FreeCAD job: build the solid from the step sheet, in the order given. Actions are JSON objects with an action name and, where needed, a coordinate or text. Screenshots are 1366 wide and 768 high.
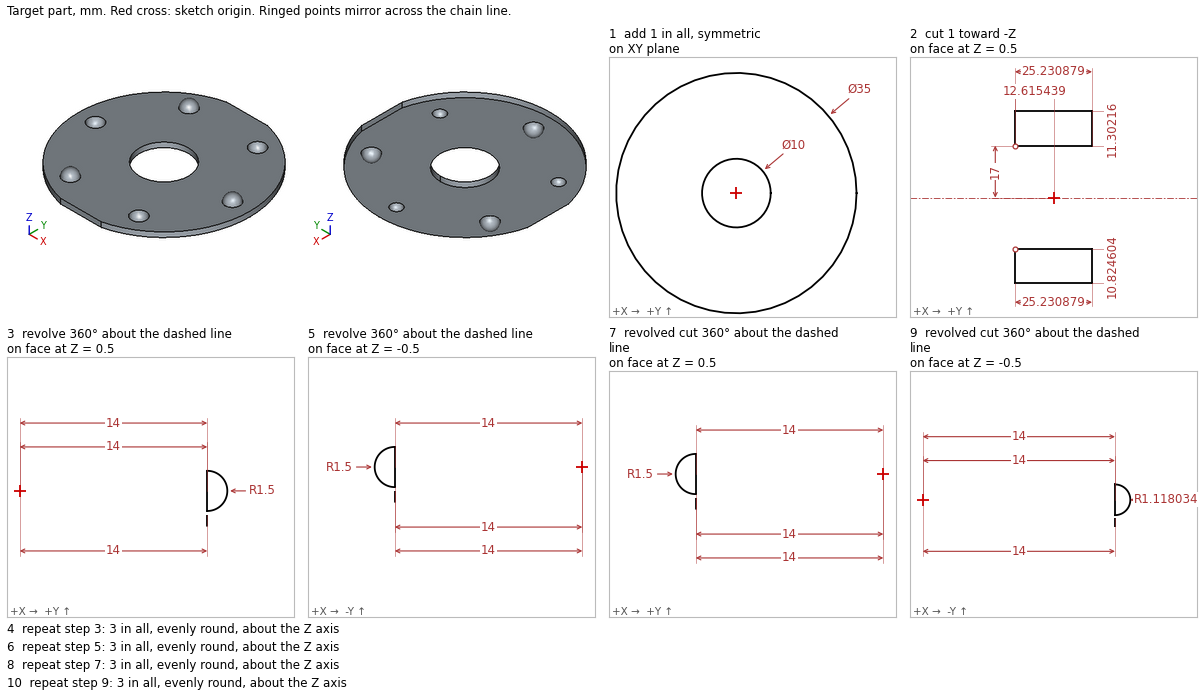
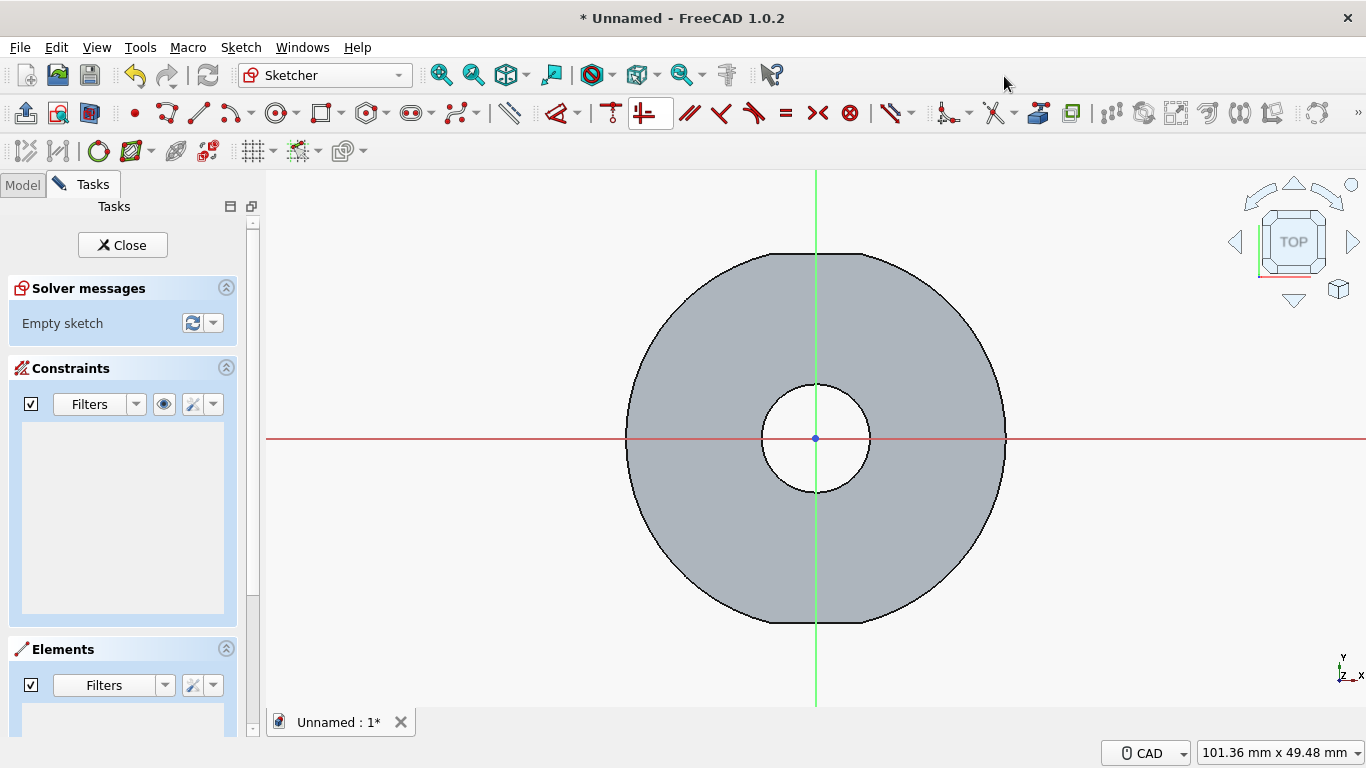
{"action": "scroll", "coordinate": [1012, 446], "scroll_direction": "up", "scroll_amount": 10}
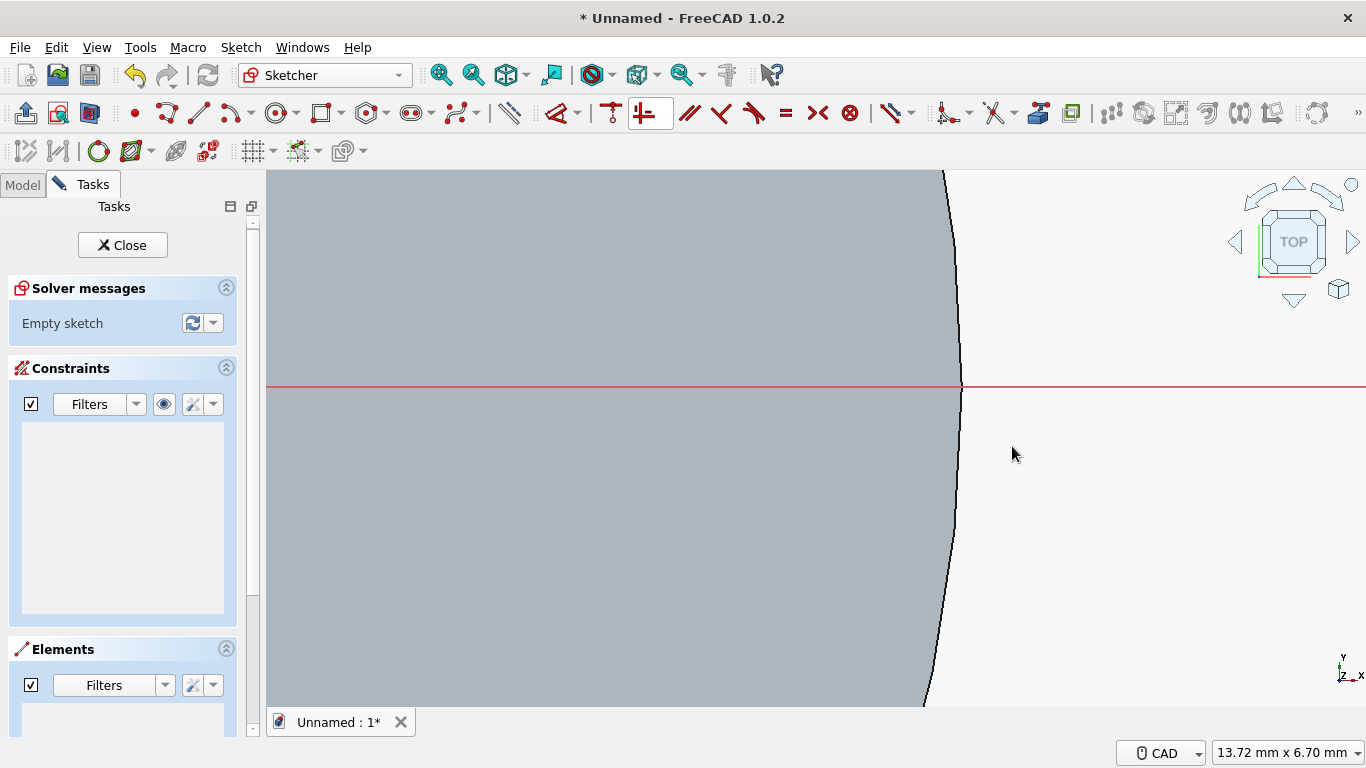
{"action": "key", "text": "g l"}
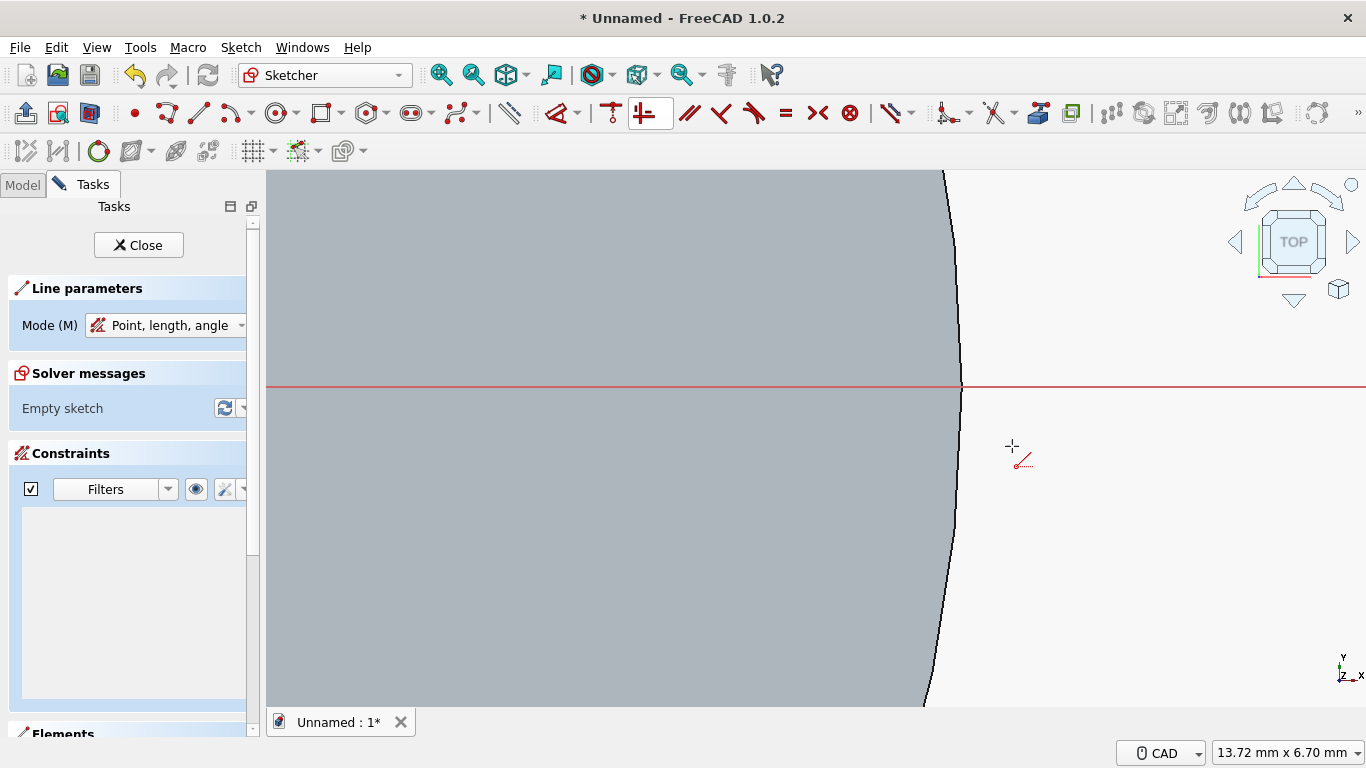
{"action": "left_click", "coordinate": [681, 267]}
{"action": "left_click", "coordinate": [681, 508]}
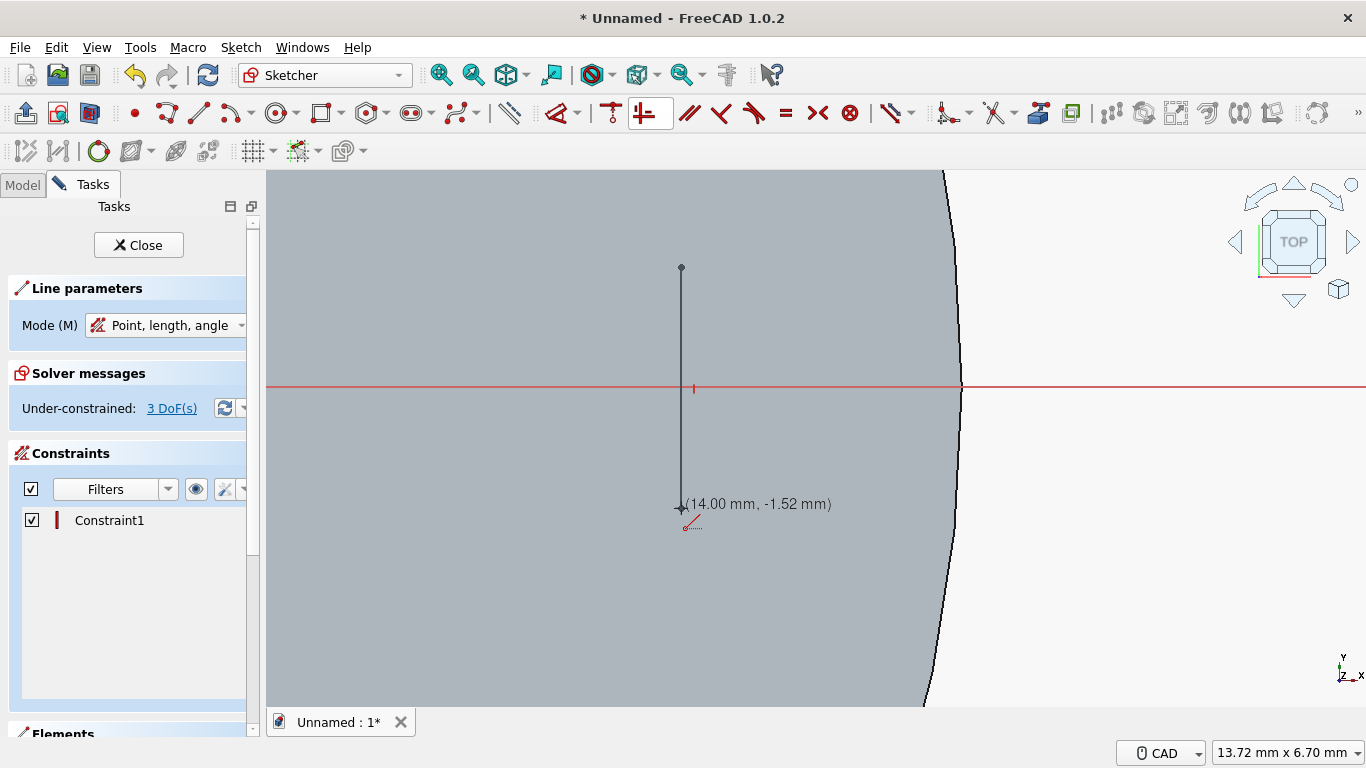
{"action": "key", "text": "g 3 a"}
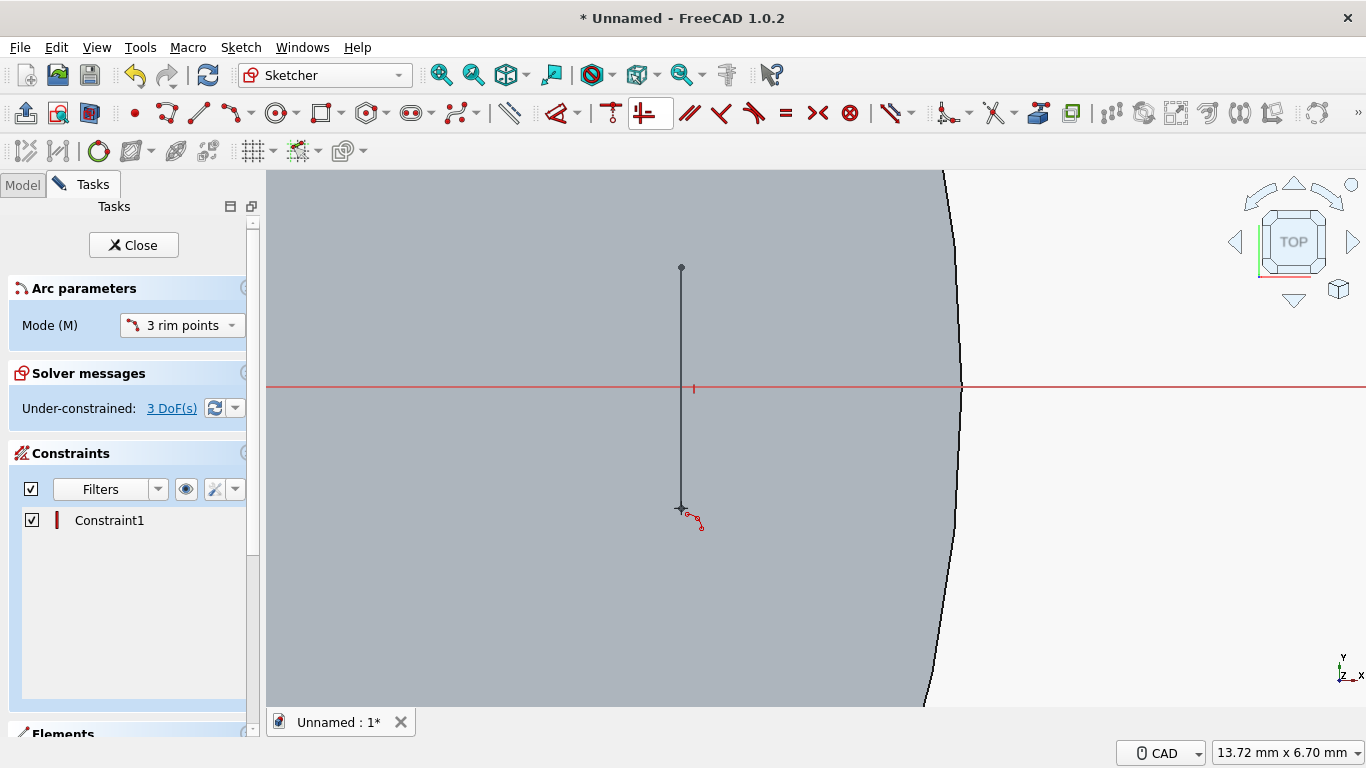
{"action": "left_click", "coordinate": [681, 509]}
{"action": "left_click", "coordinate": [681, 268]}
{"action": "left_click", "coordinate": [795, 424]}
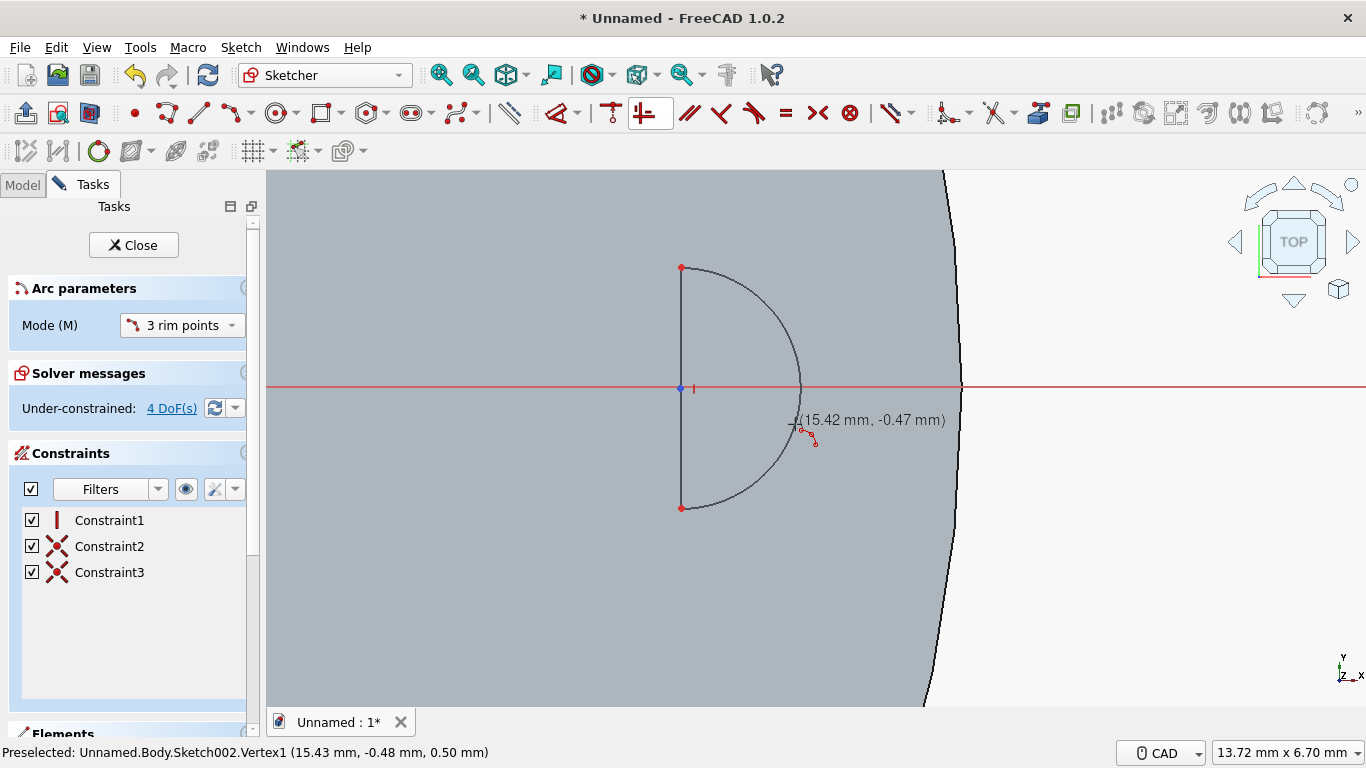
{"action": "key", "text": "g l"}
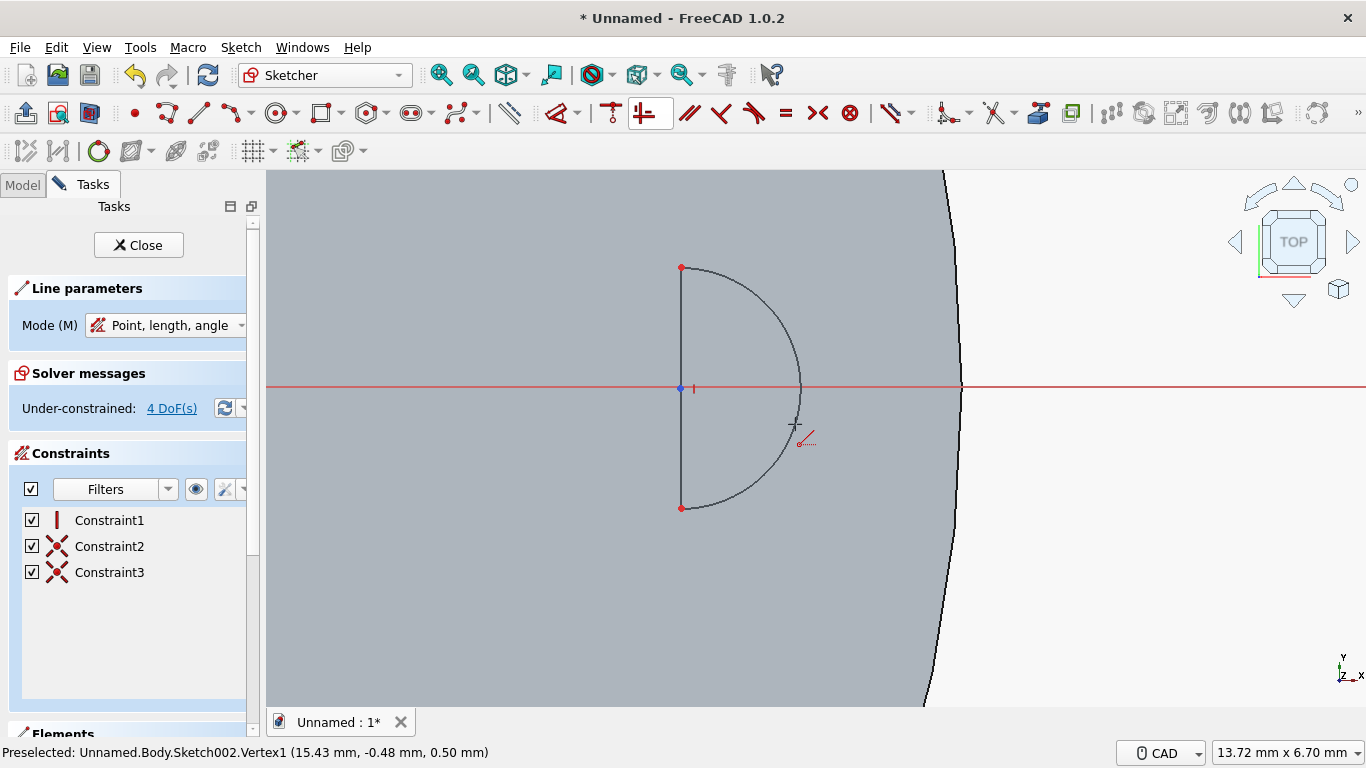
{"action": "left_click", "coordinate": [681, 532]}
{"action": "left_click", "coordinate": [681, 604]}
{"action": "key", "text": "Escape"}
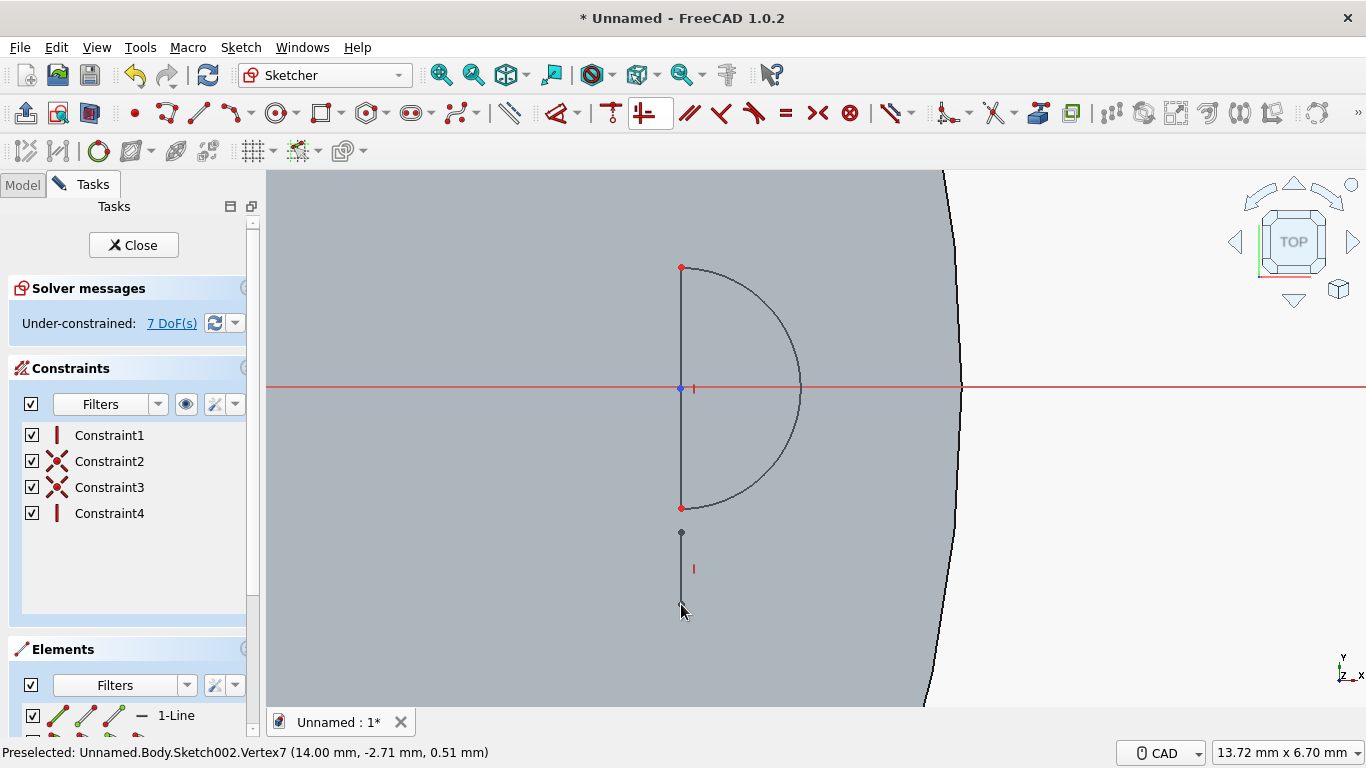
{"action": "left_click", "coordinate": [681, 555]}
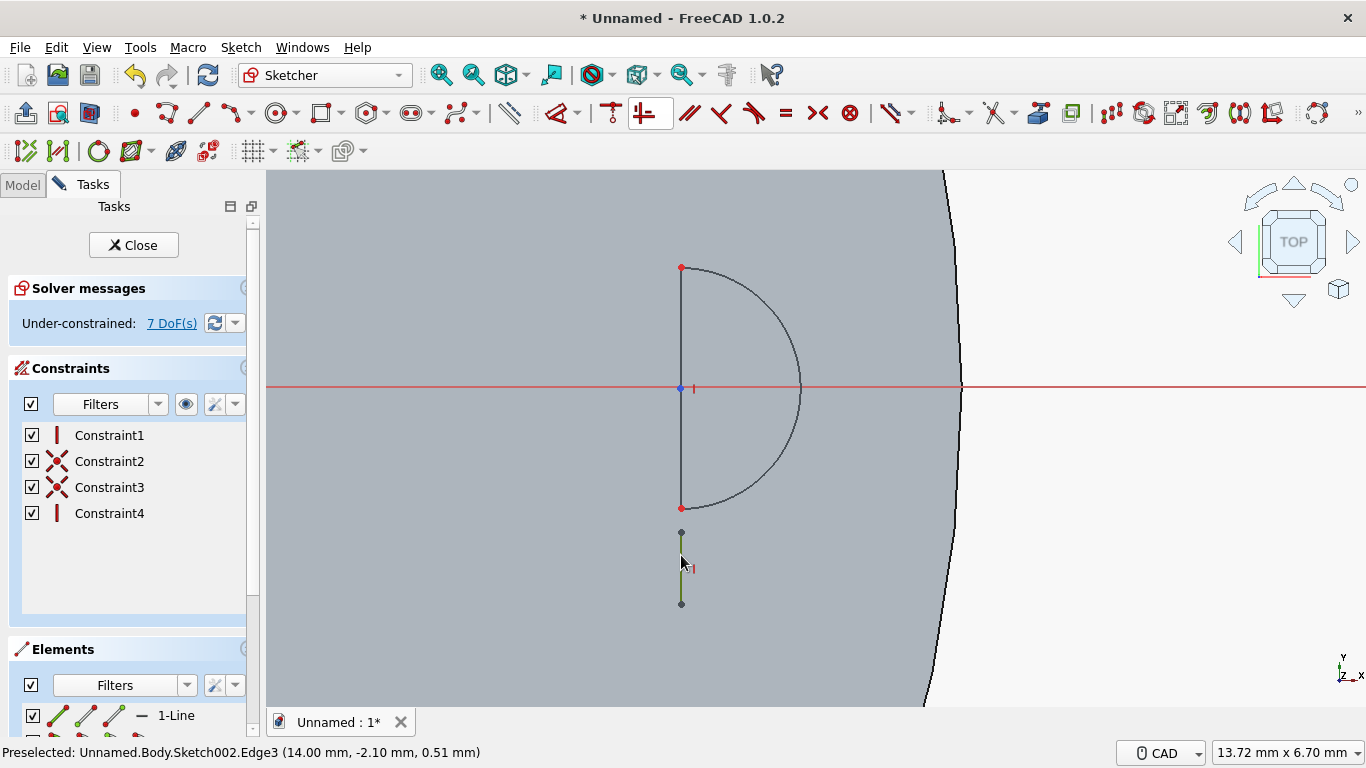
{"action": "key", "text": "g n"}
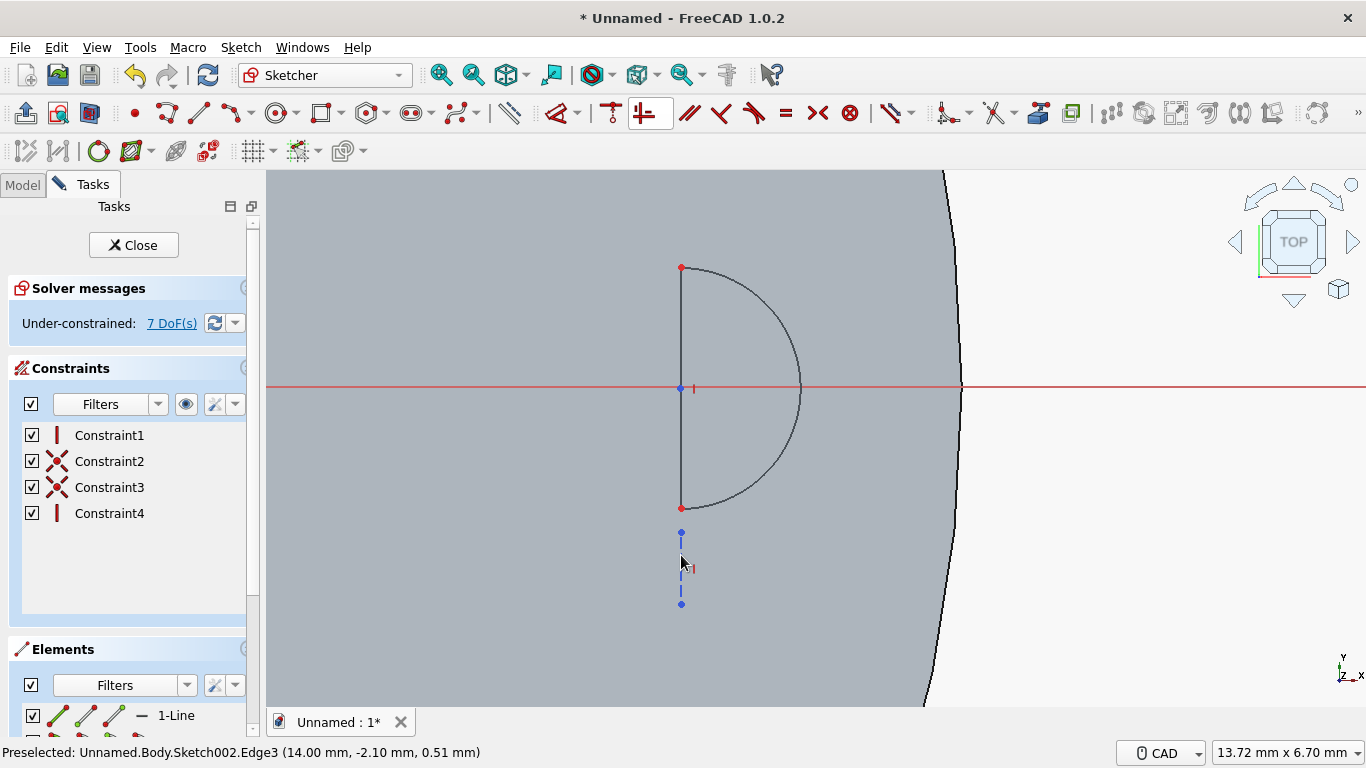
{"action": "left_click", "coordinate": [680, 388]}